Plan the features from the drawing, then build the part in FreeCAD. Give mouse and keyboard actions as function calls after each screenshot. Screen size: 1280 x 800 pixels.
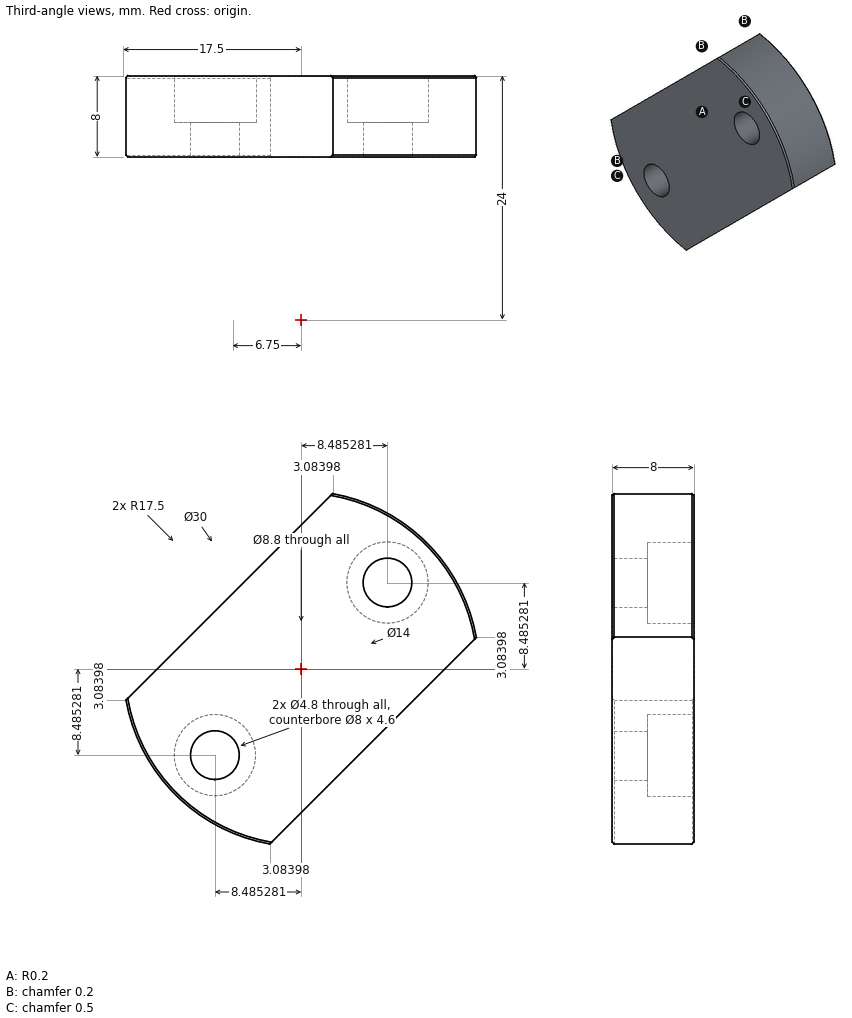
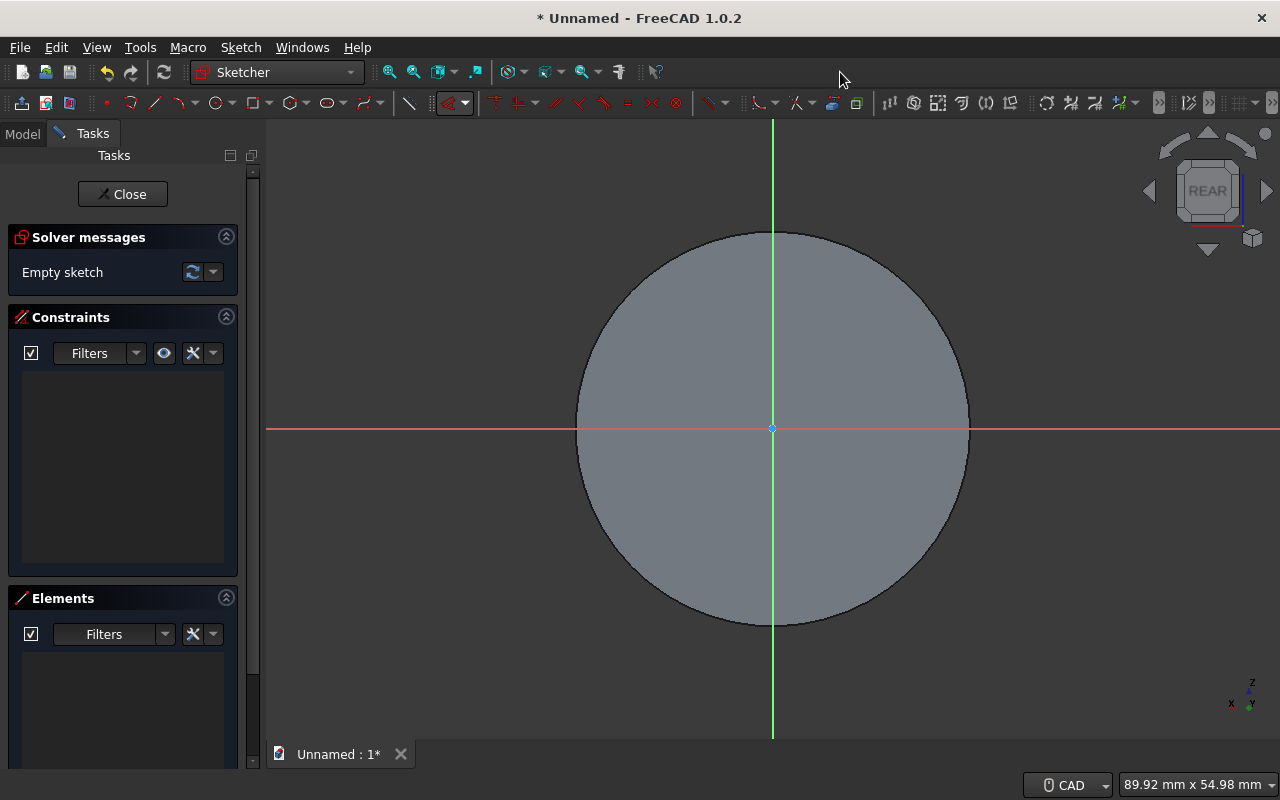
scroll(795, 429, up, 7)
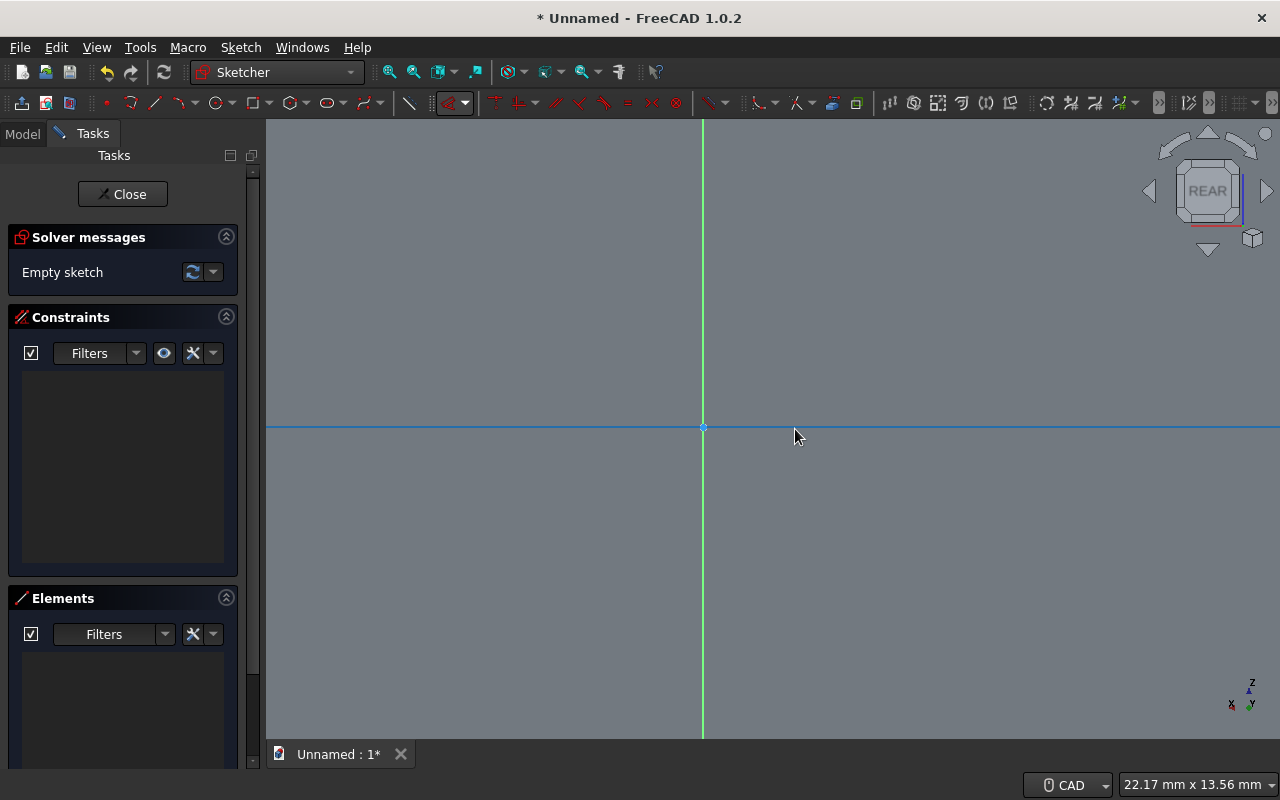
click(216, 104)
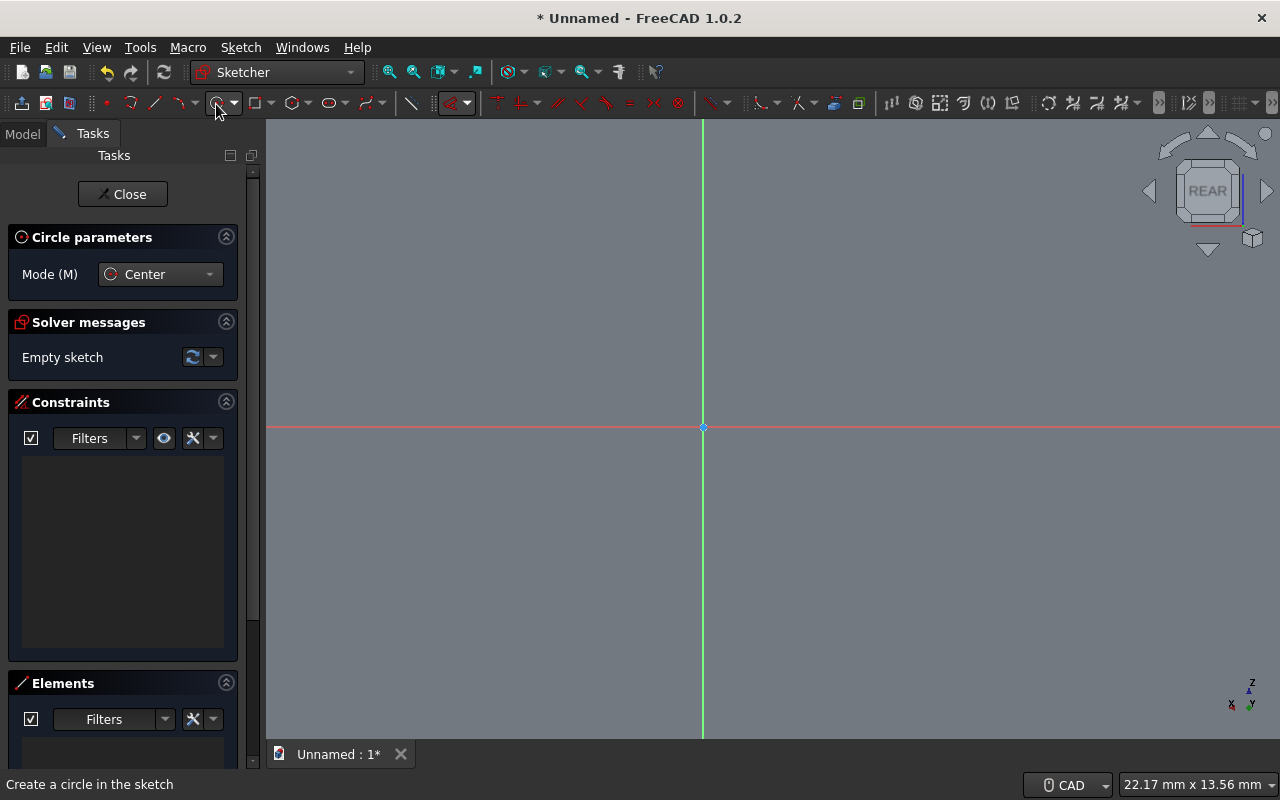
click(703, 427)
move(846, 285)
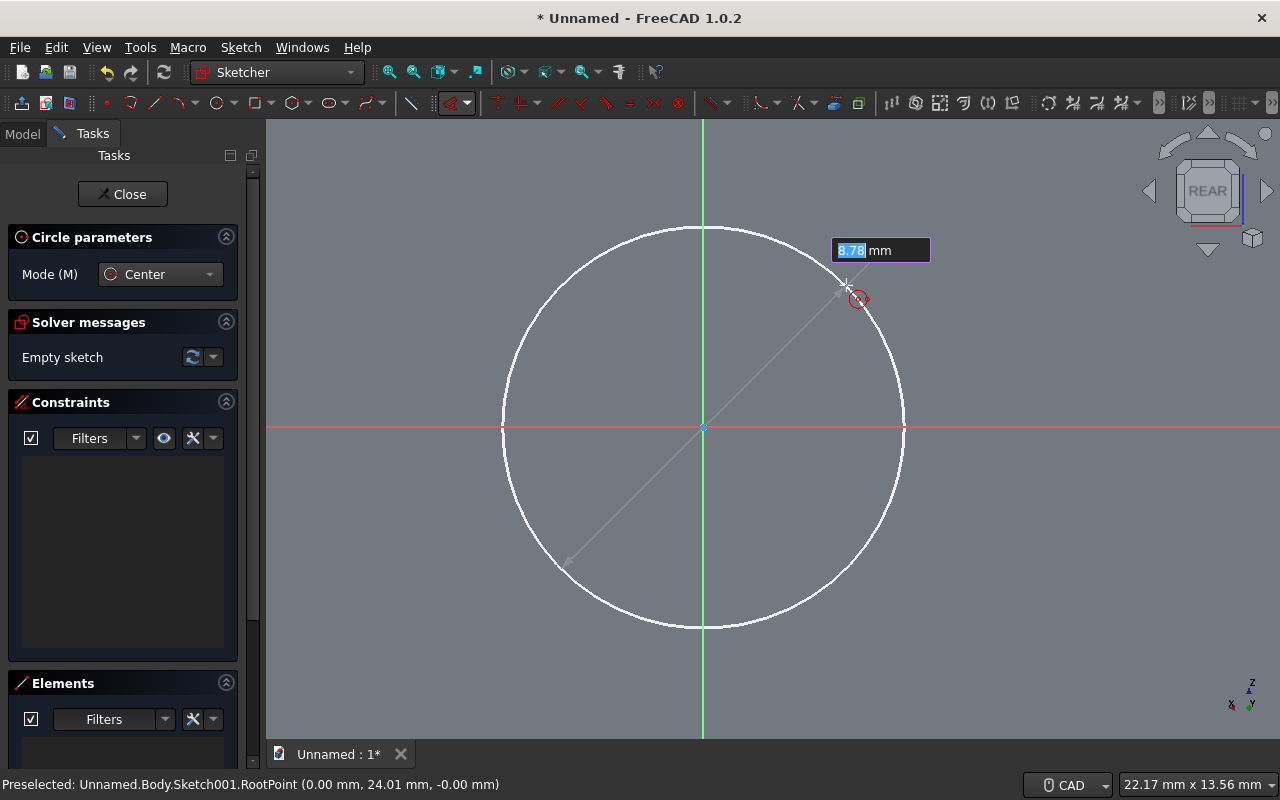
text(8.8)
key(Return)
key(Escape)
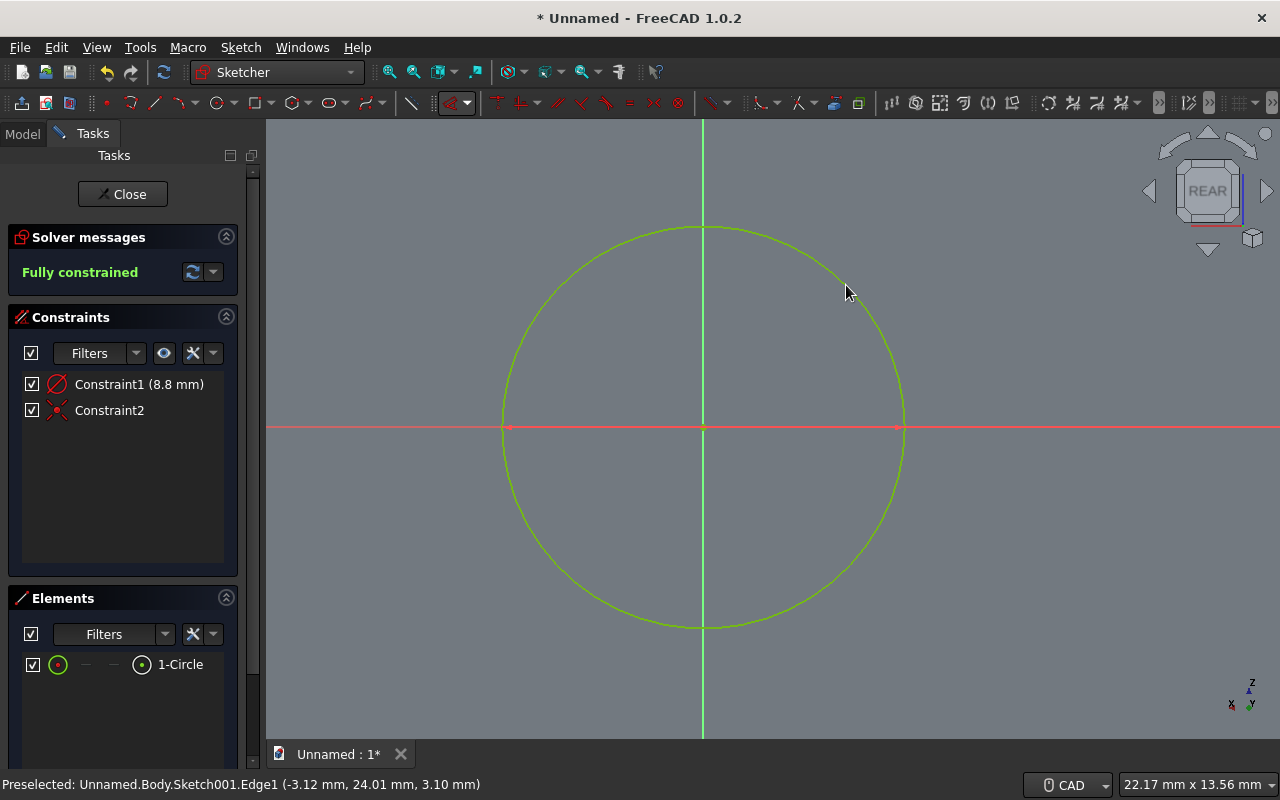
click(123, 194)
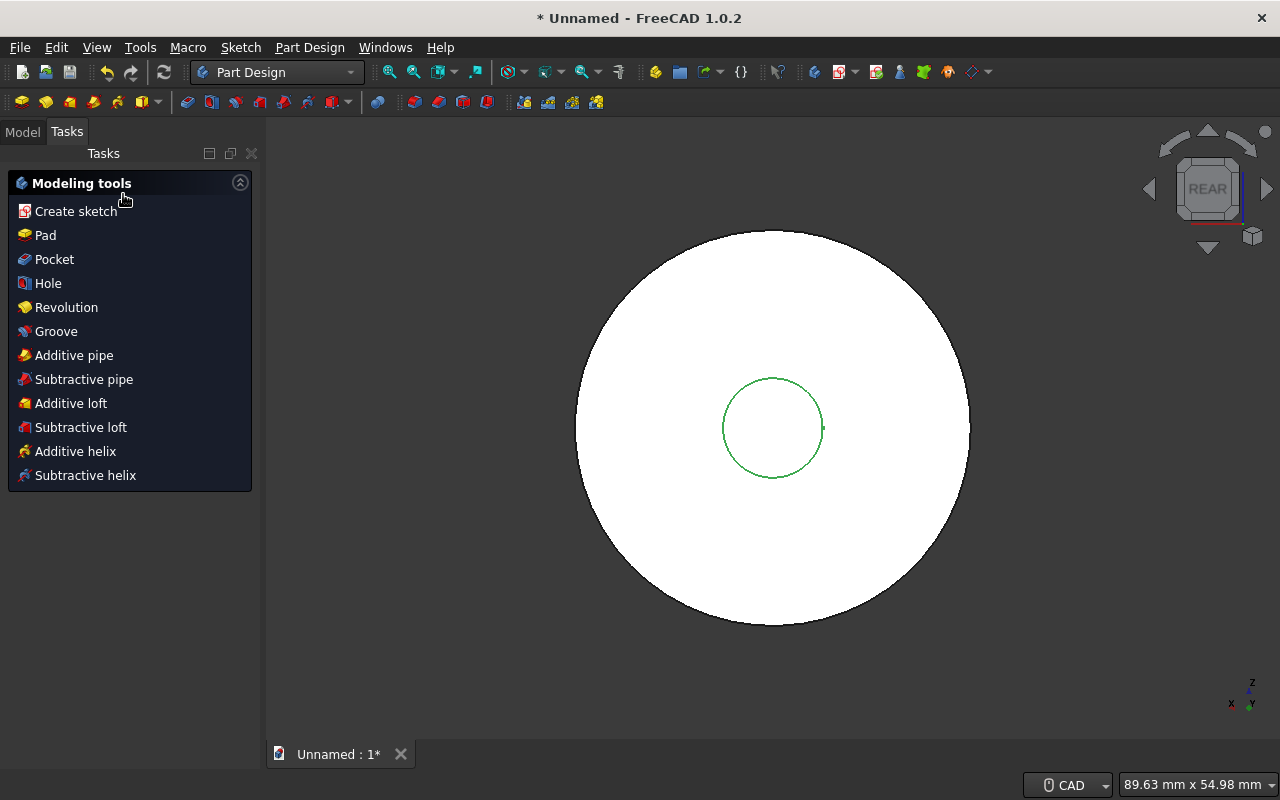
click(212, 102)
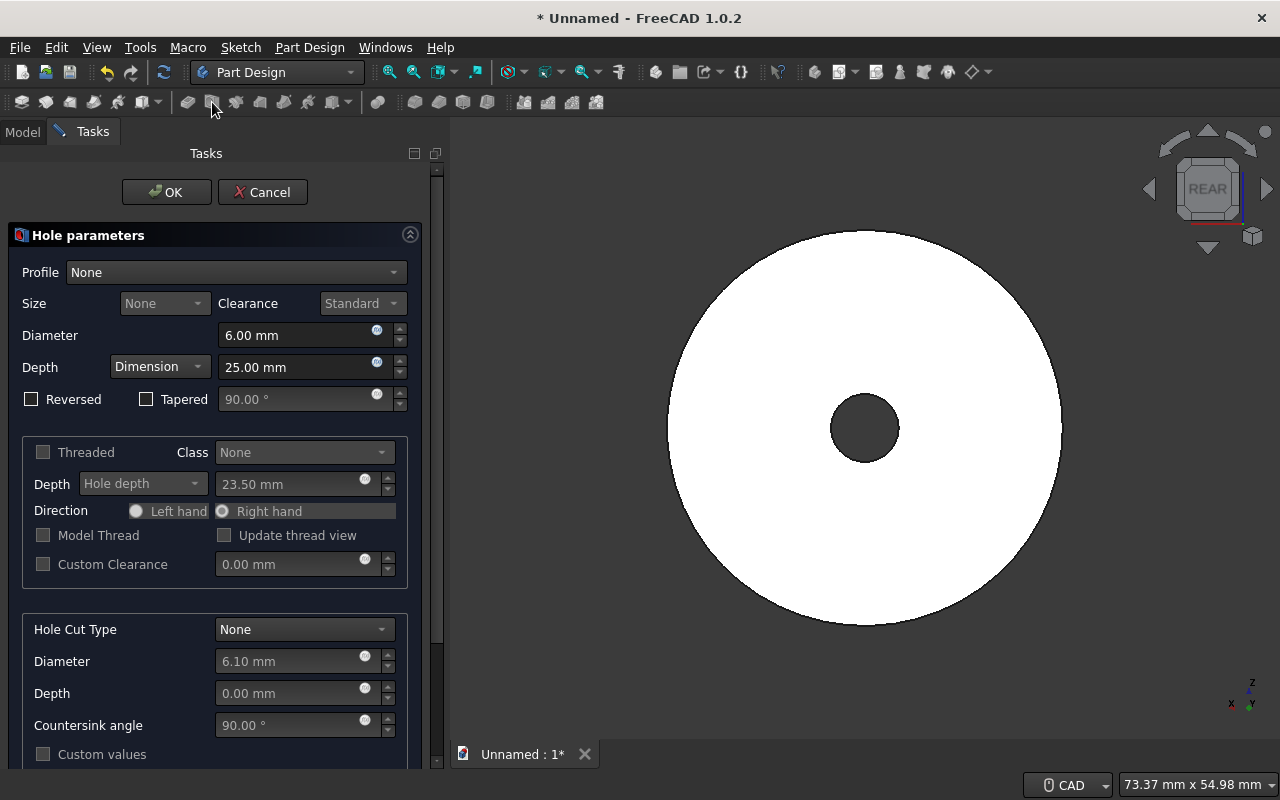
triple_click(305, 335)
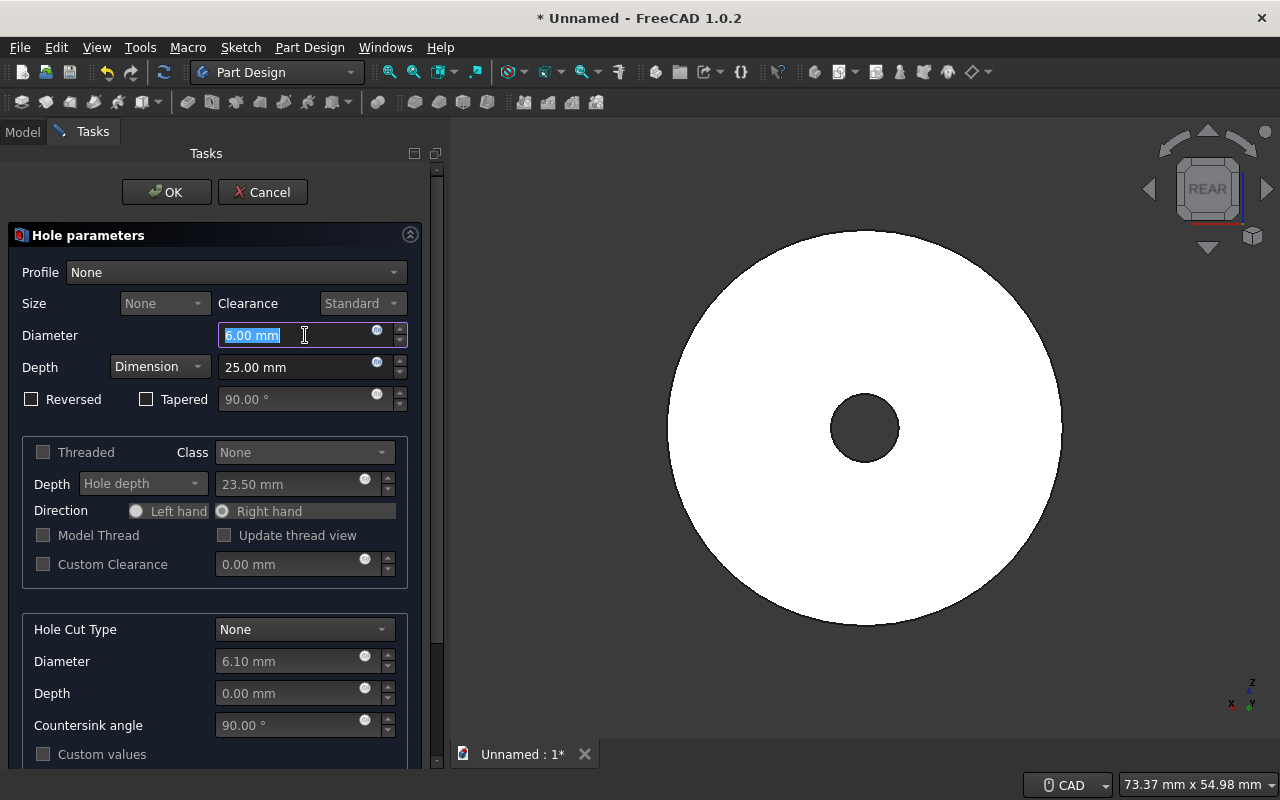
text(8.8)
key(Tab)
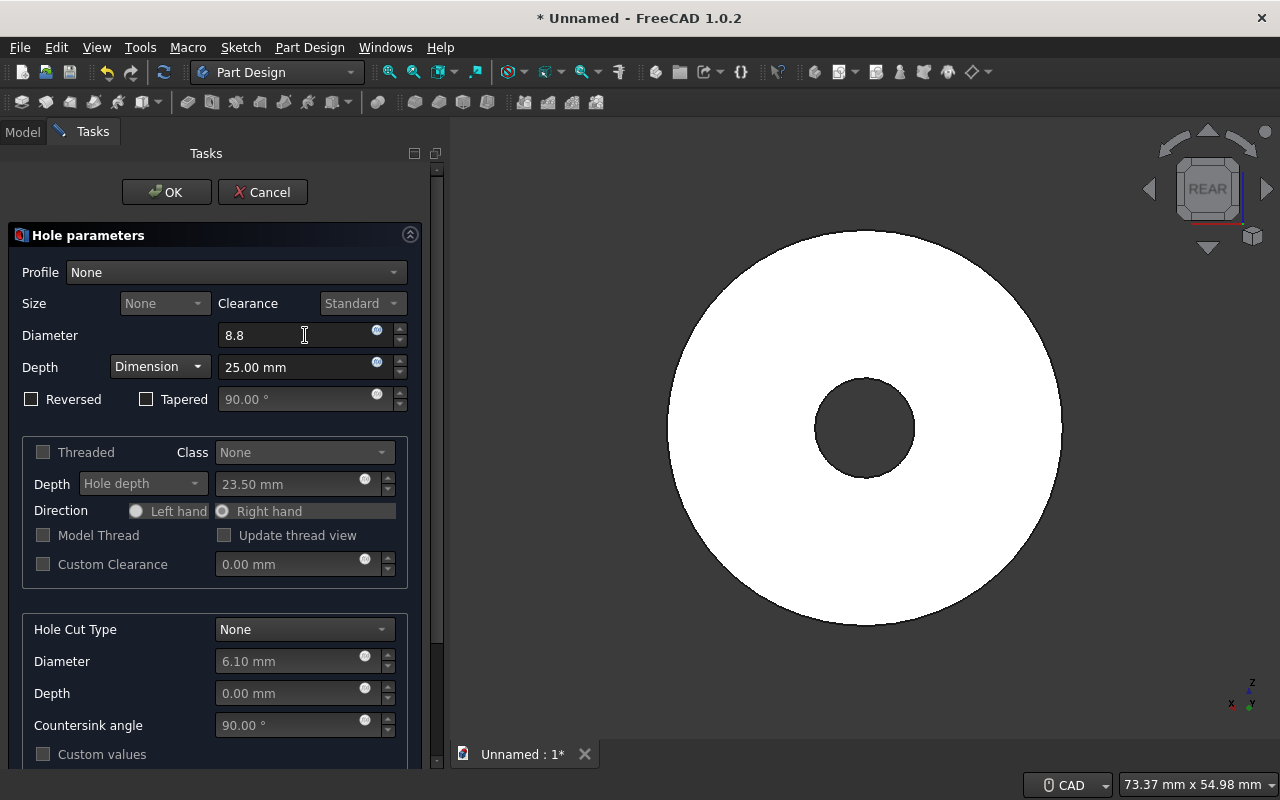
click(161, 366)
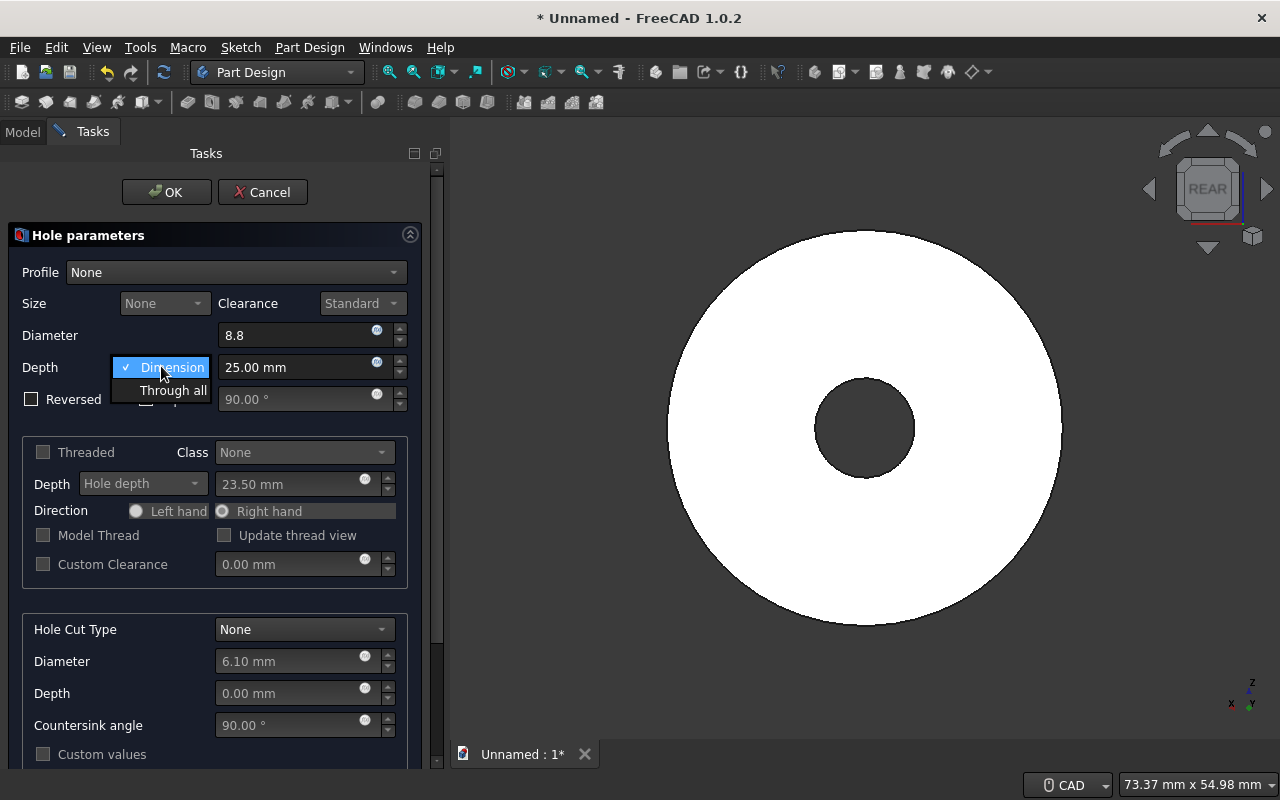
click(160, 390)